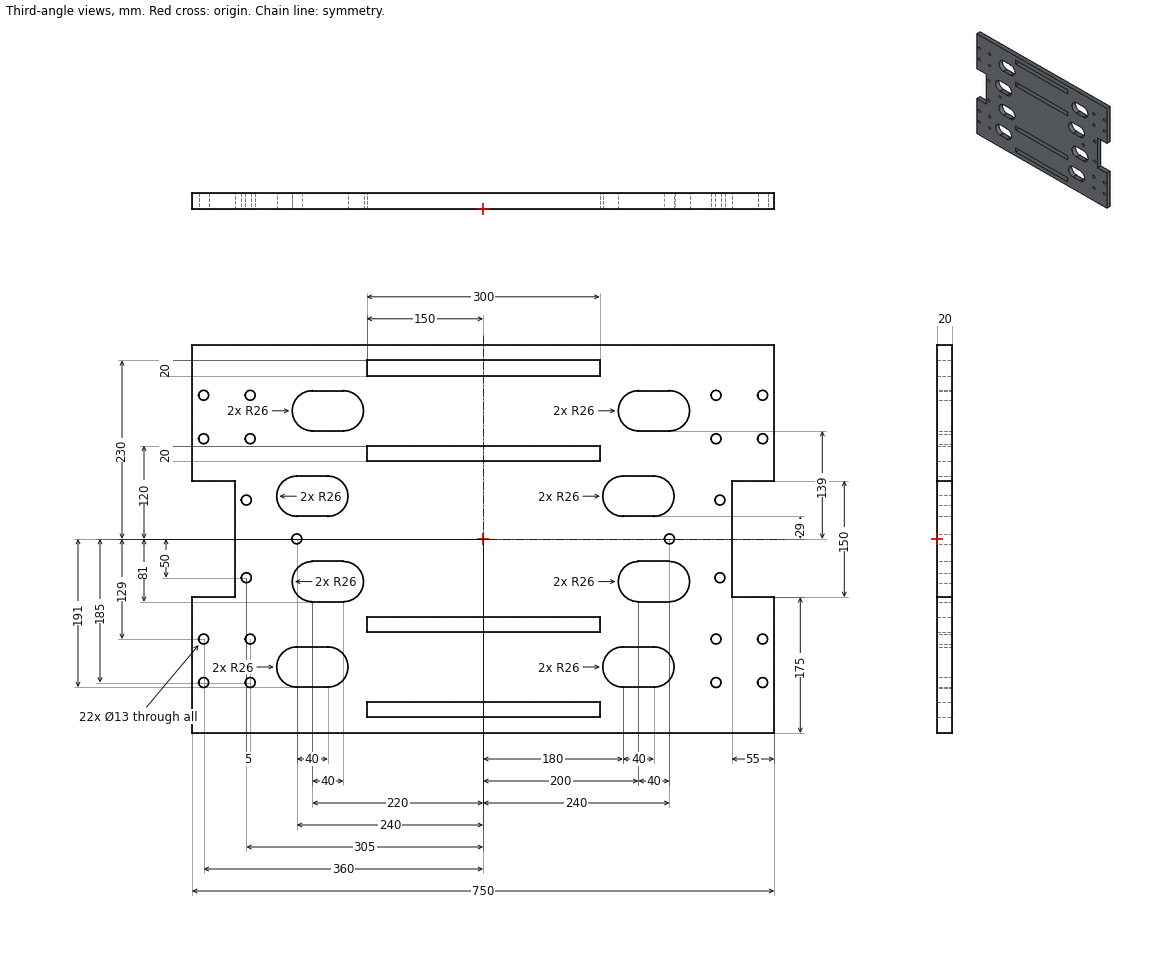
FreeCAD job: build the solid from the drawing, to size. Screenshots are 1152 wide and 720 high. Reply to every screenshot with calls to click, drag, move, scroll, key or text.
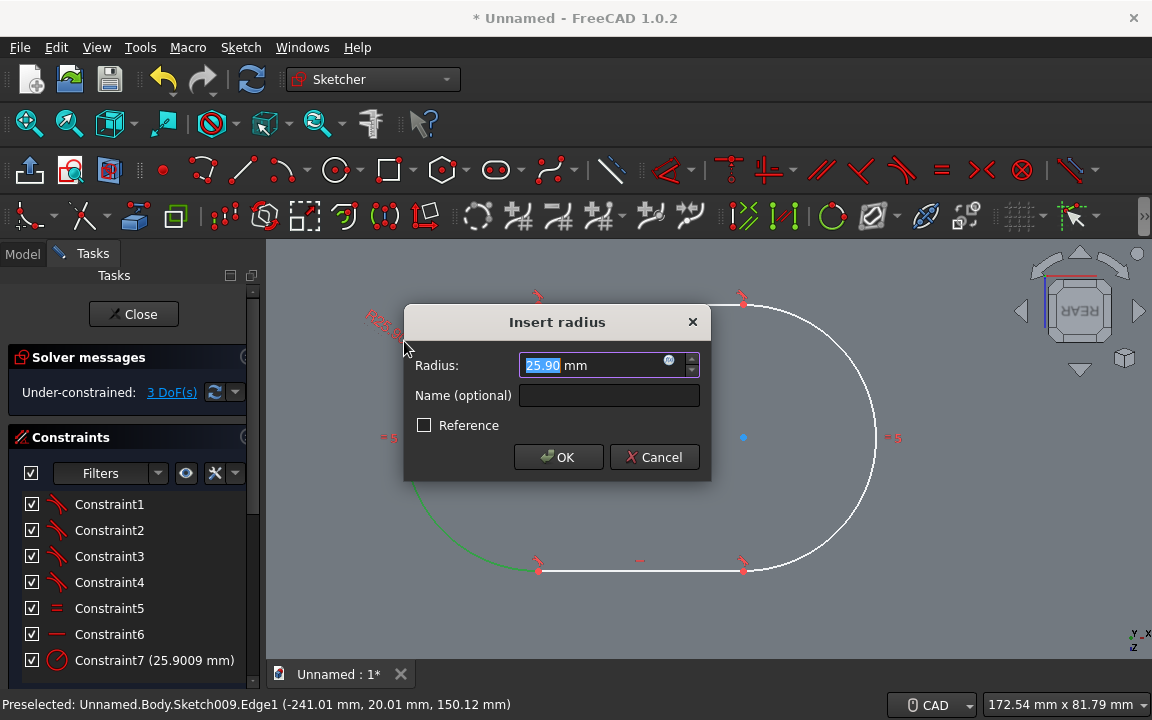
text(26)
key(Return)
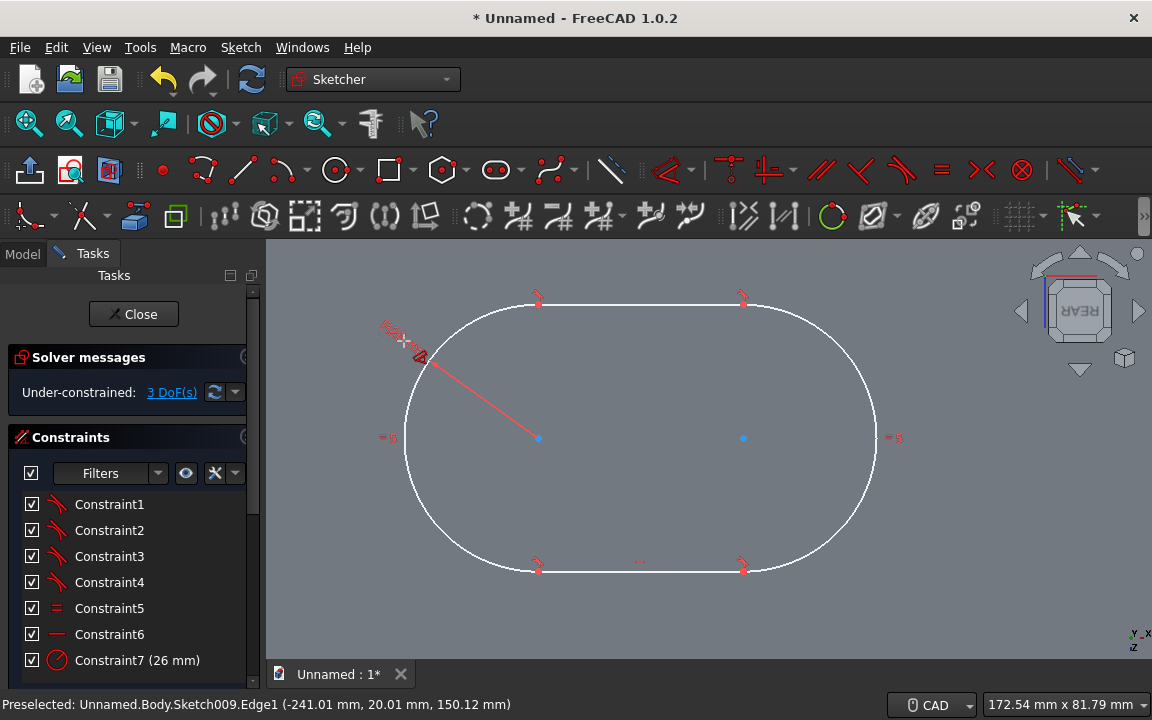
click(600, 305)
click(641, 271)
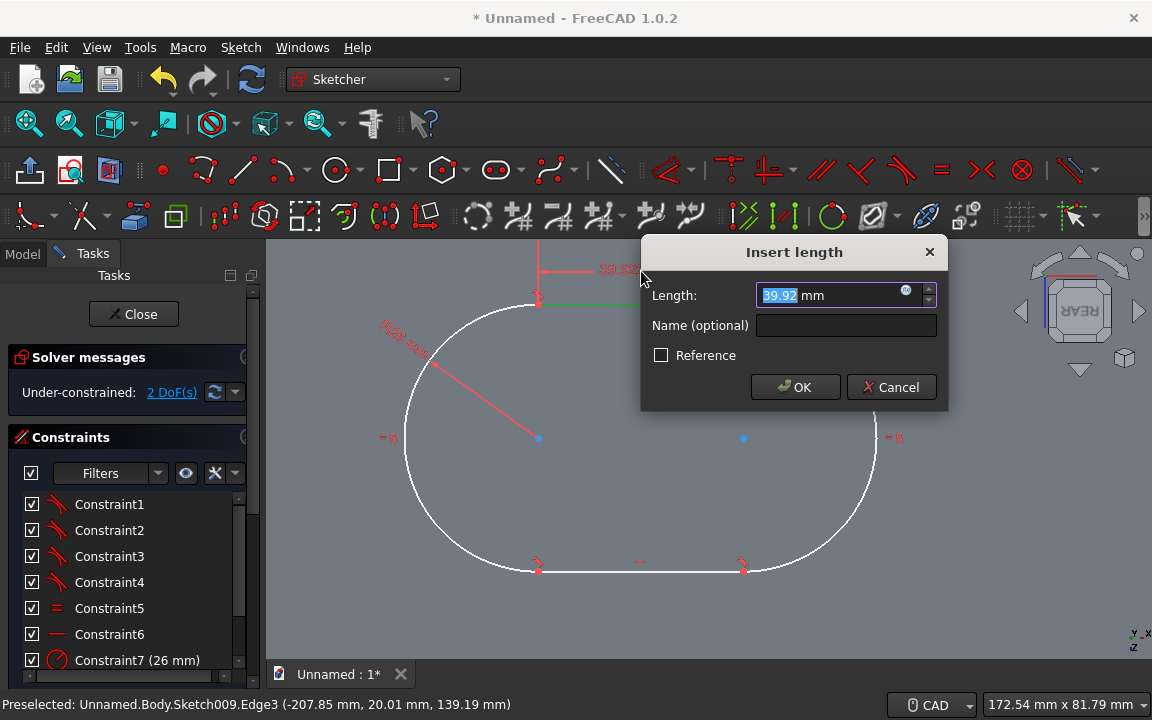
text(40)
key(Return)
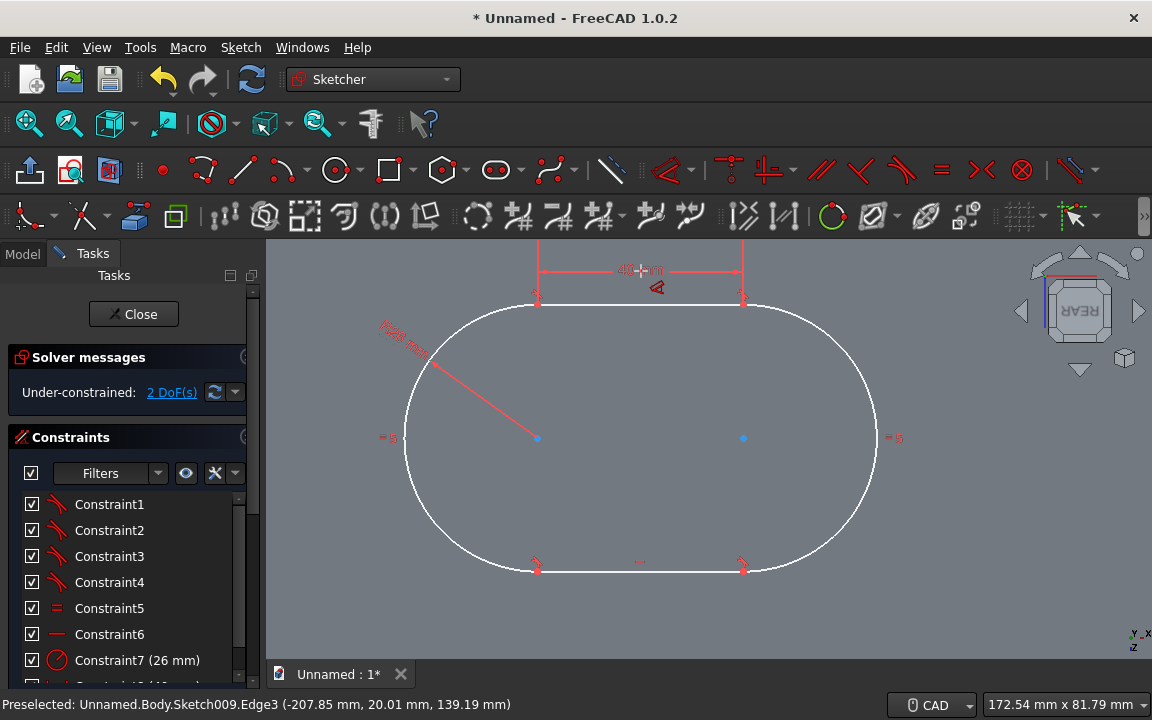
click(538, 305)
click(762, 339)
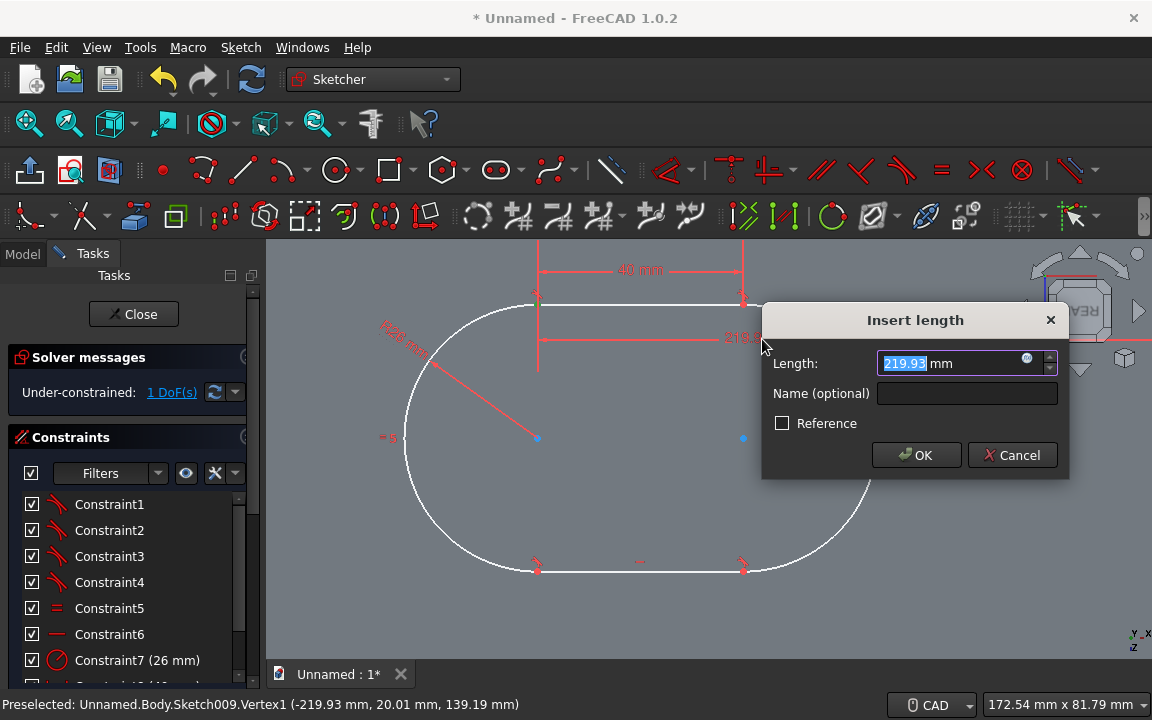
text(220)
key(Return)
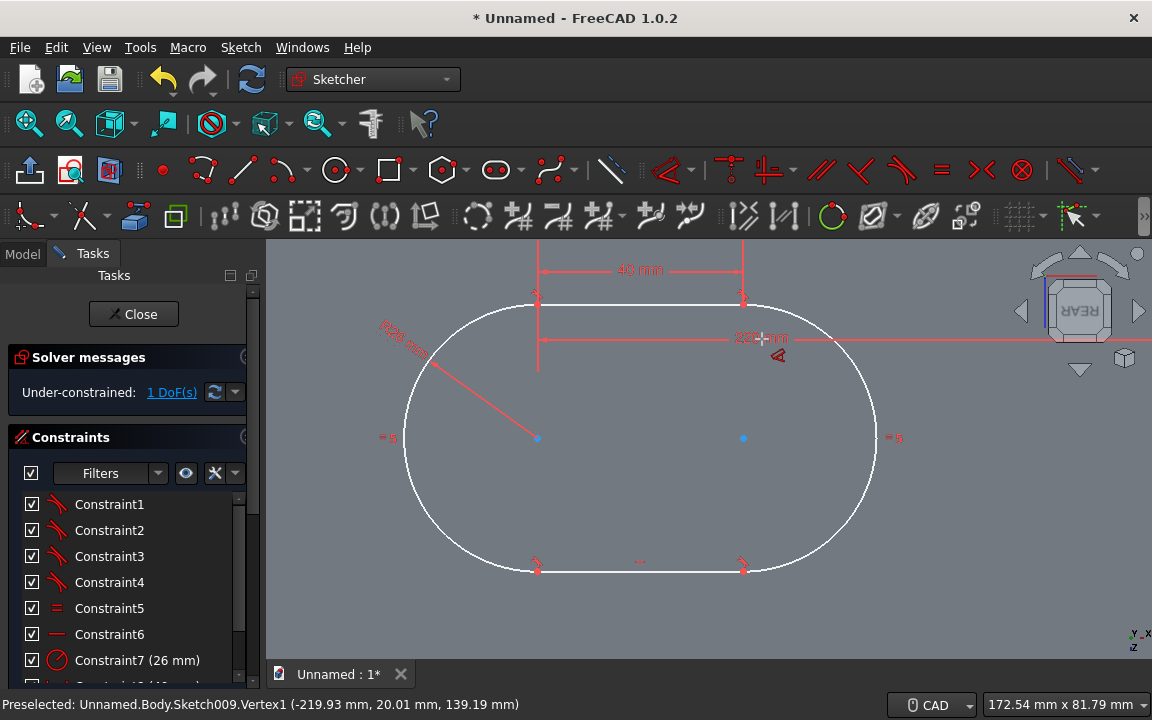
click(538, 305)
click(504, 286)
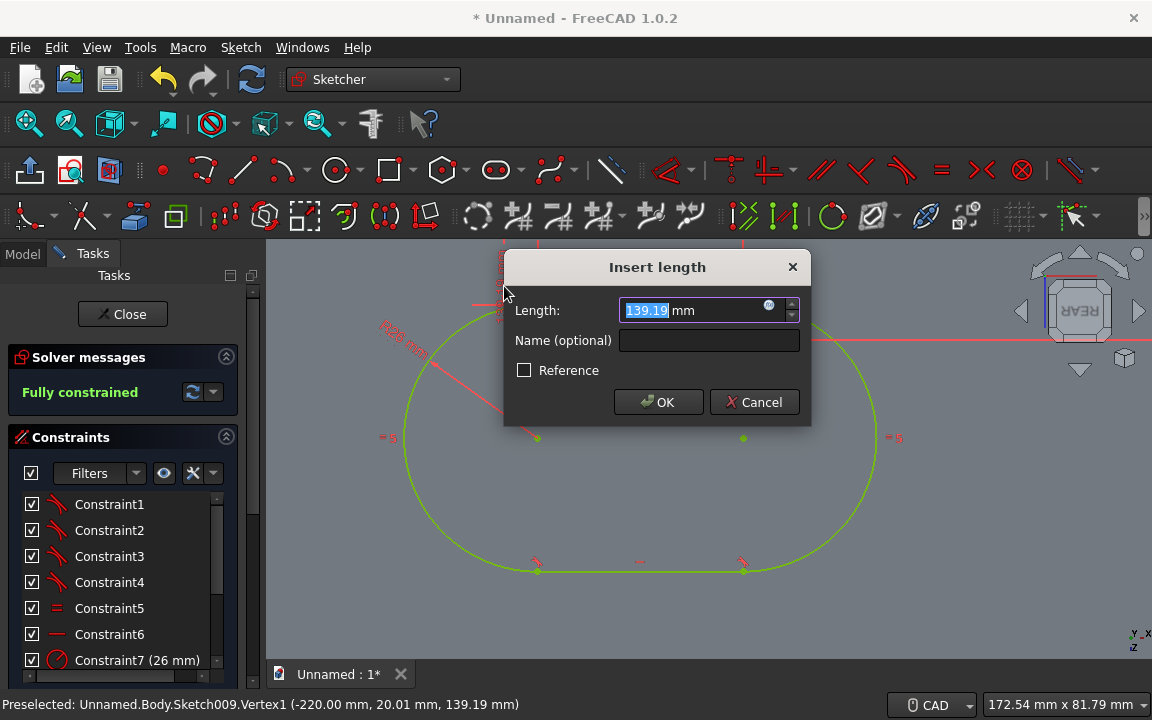
text(139)
key(Return)
key(Escape)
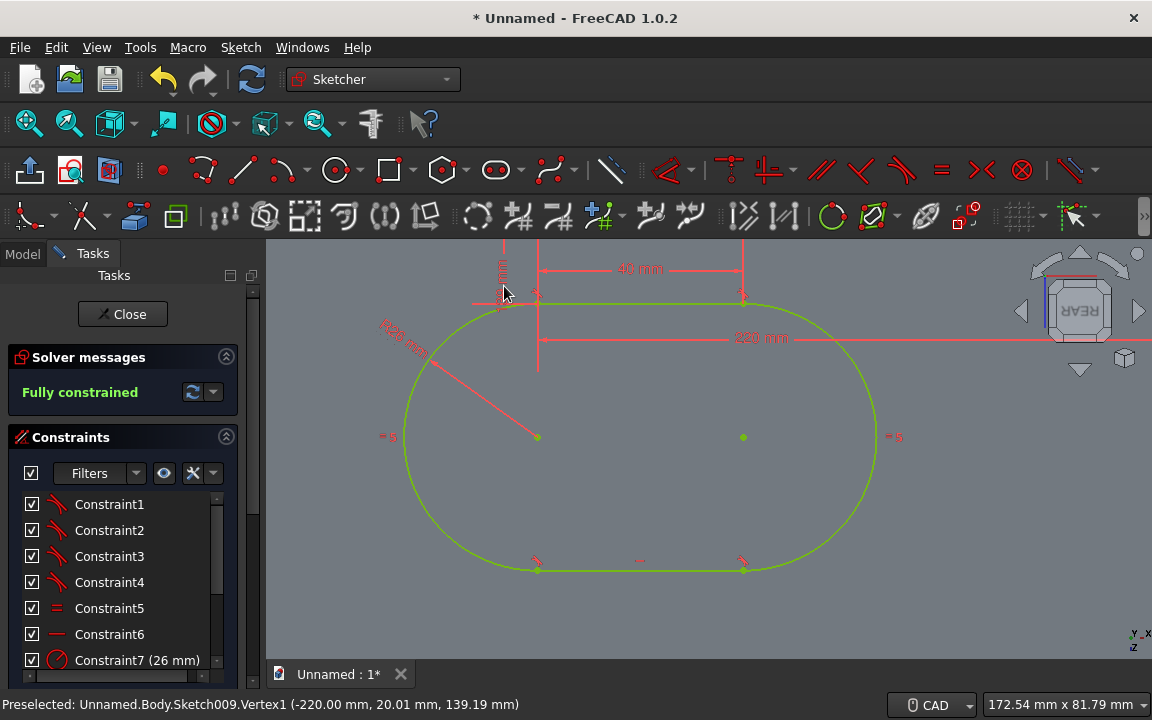
click(123, 314)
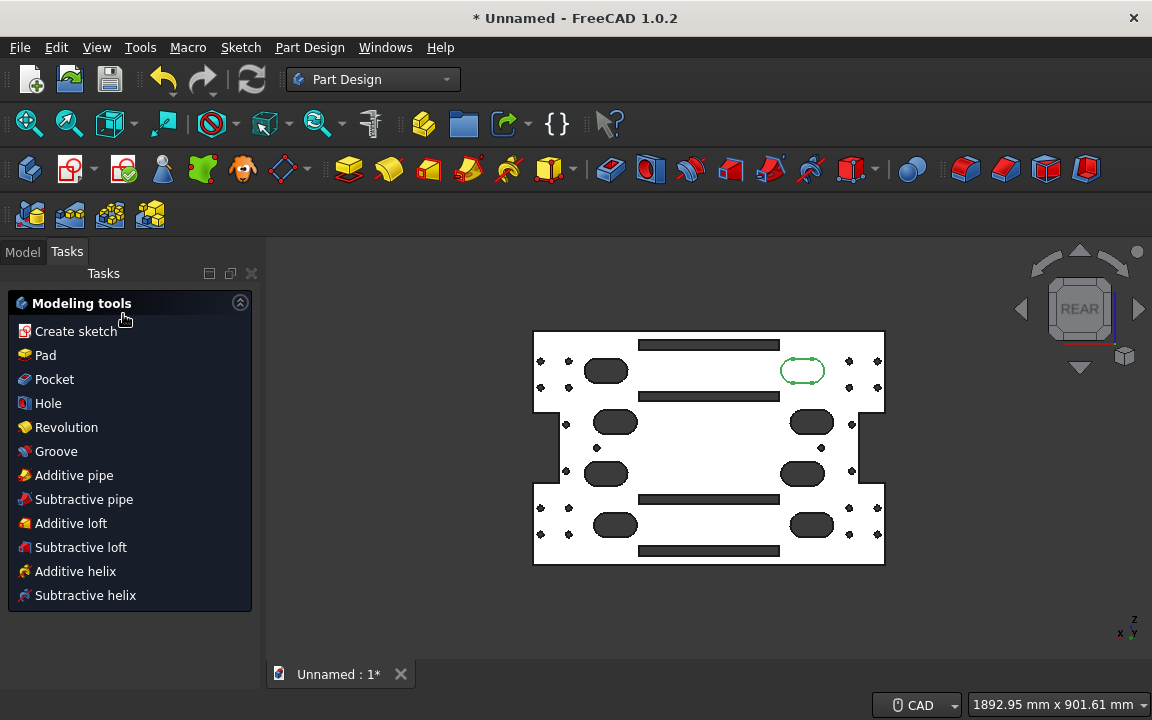
click(612, 170)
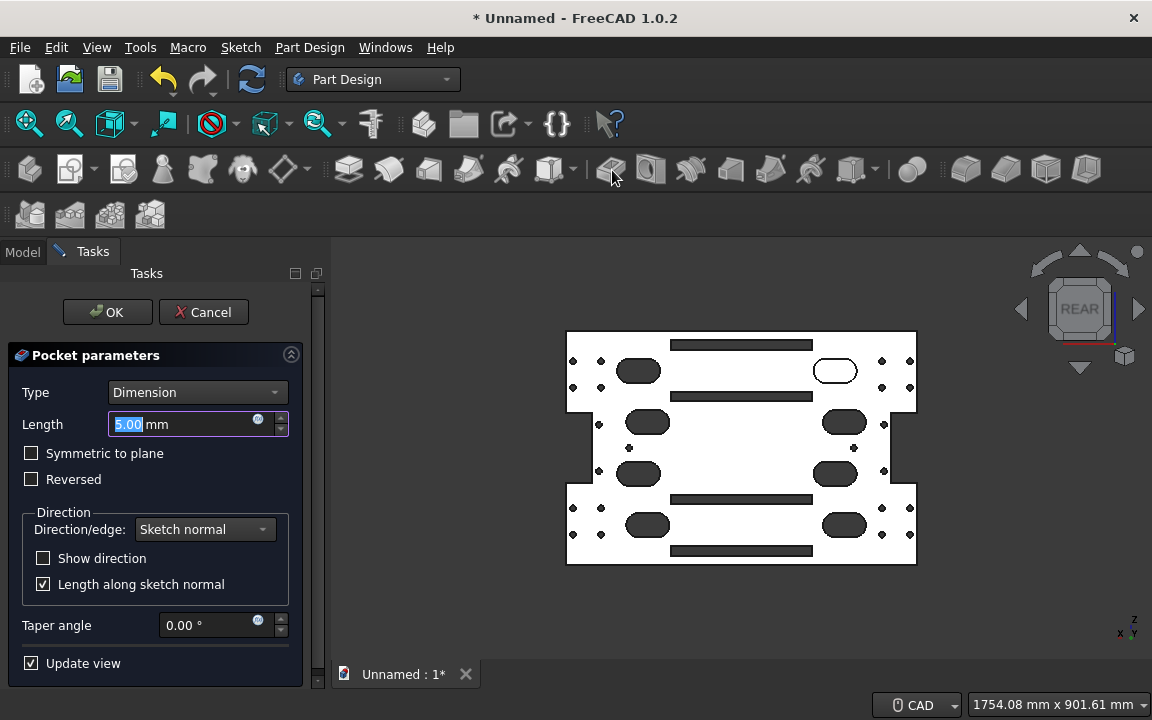
click(198, 392)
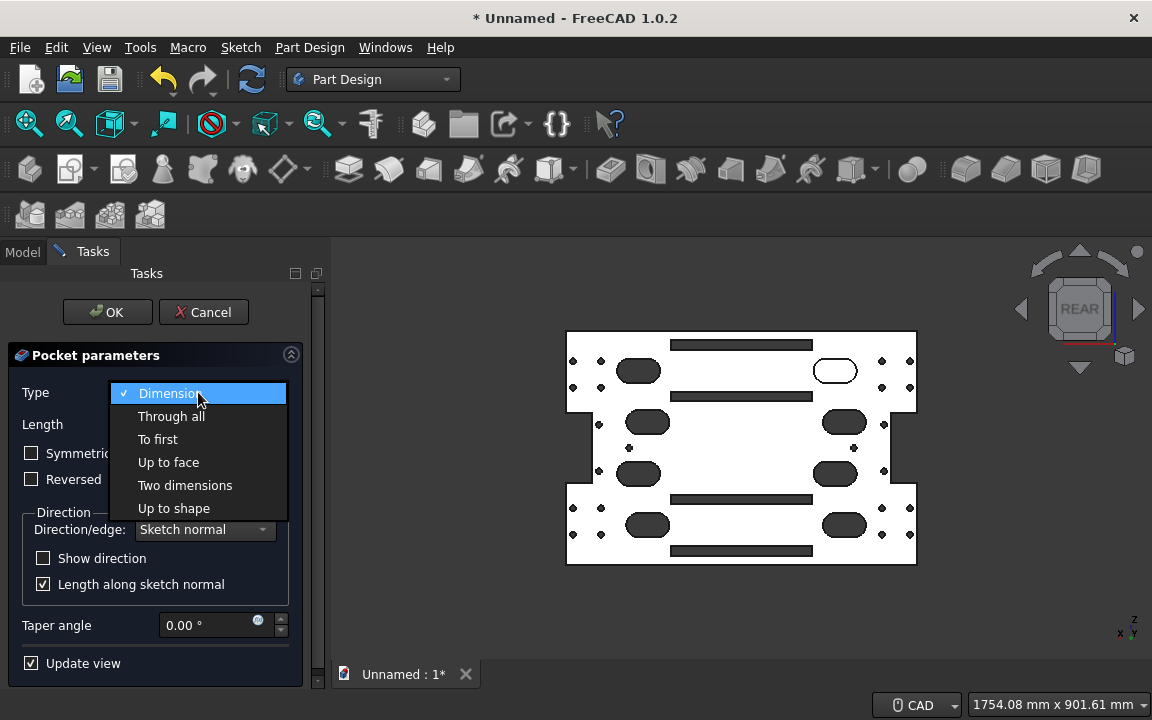
click(198, 440)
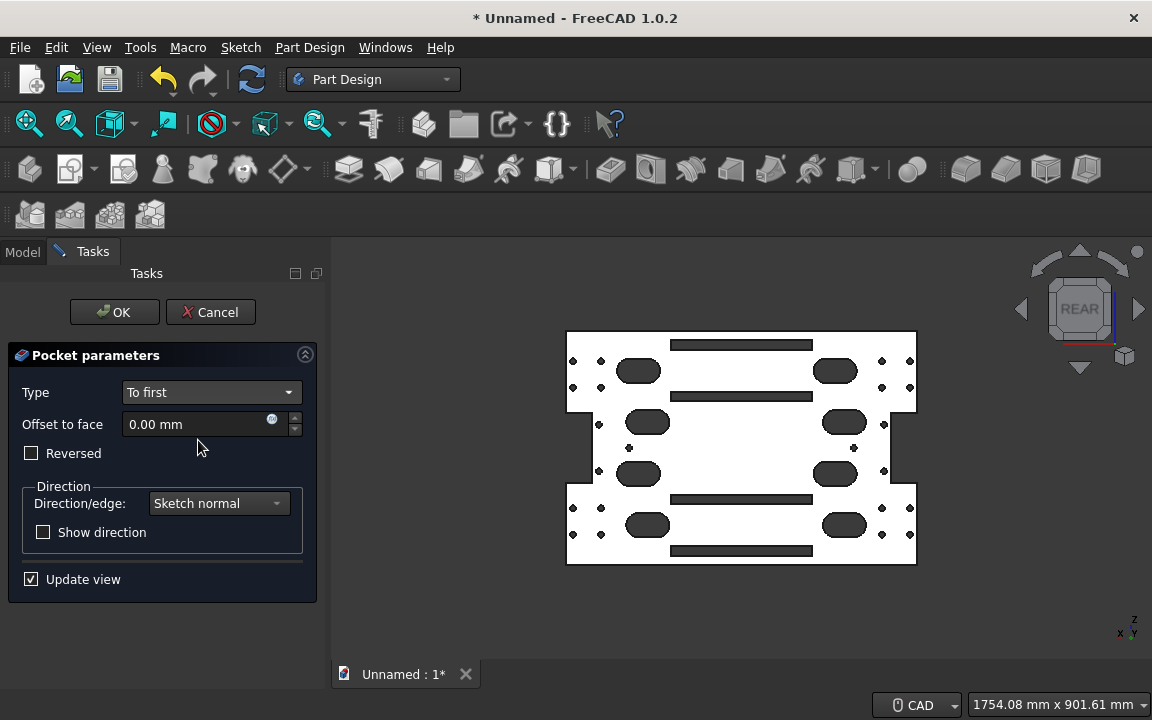
click(115, 312)